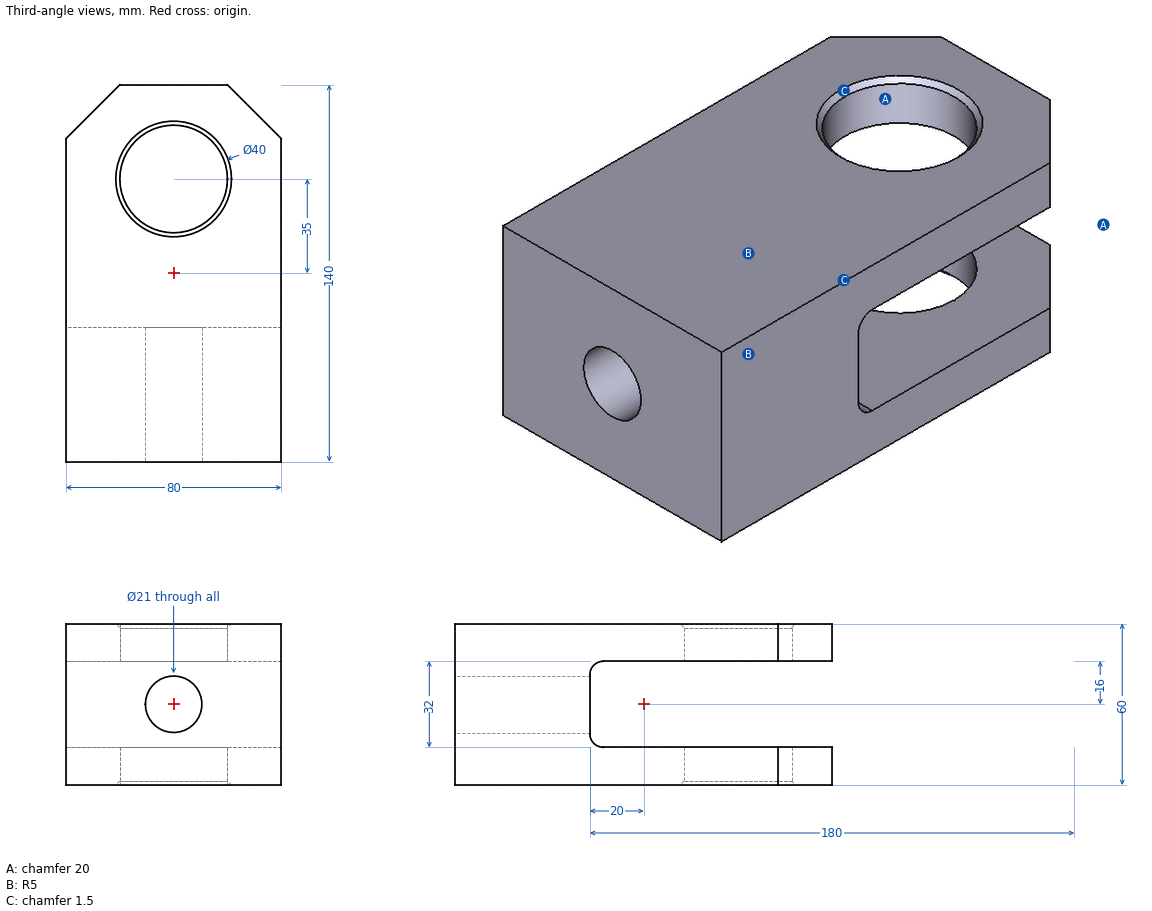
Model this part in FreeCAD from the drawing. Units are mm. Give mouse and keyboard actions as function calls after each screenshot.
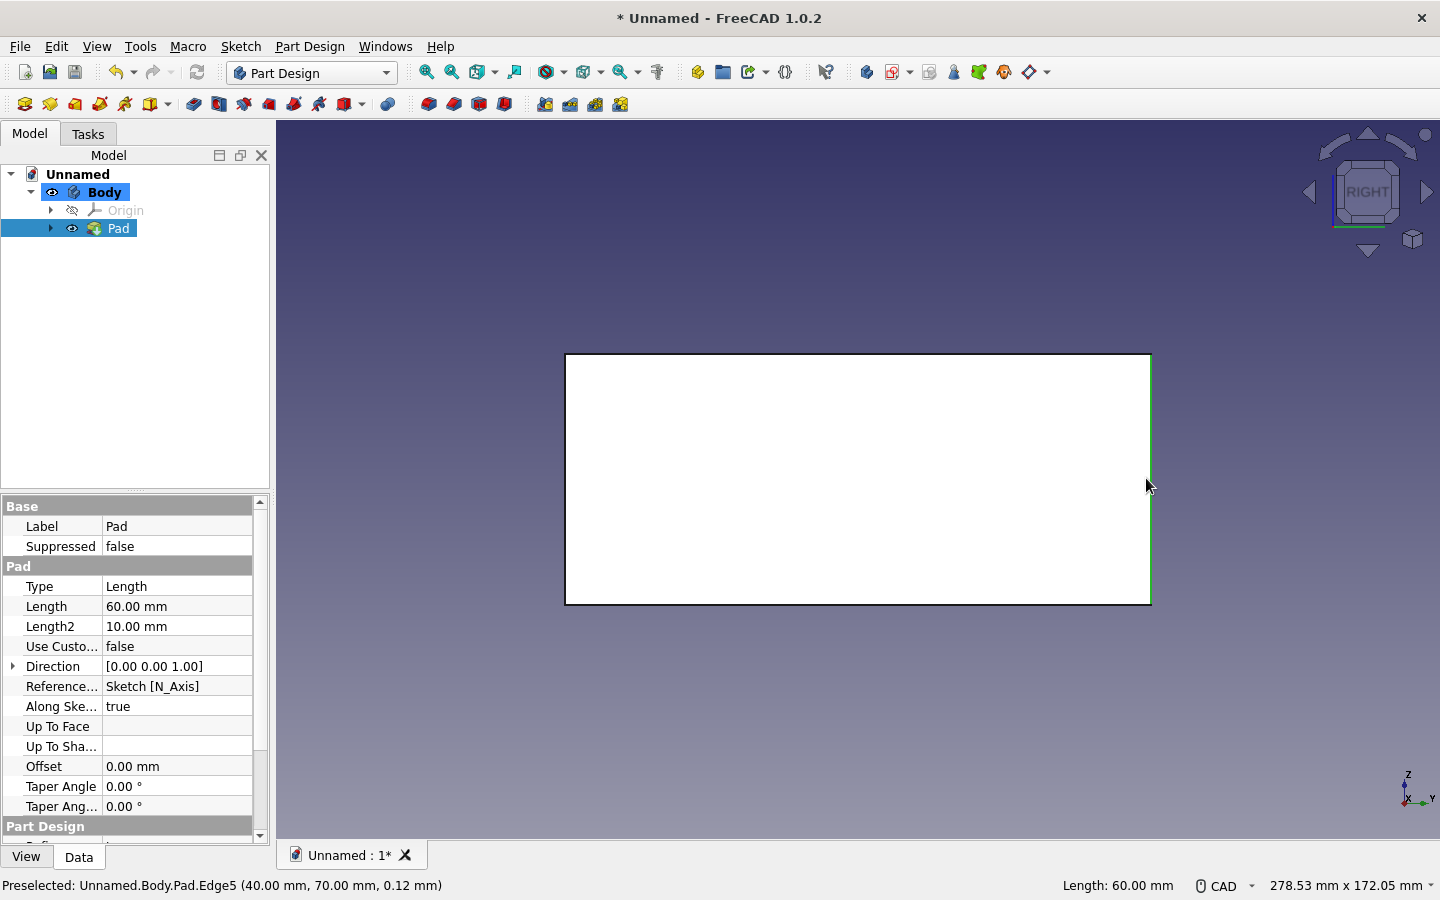
key(5)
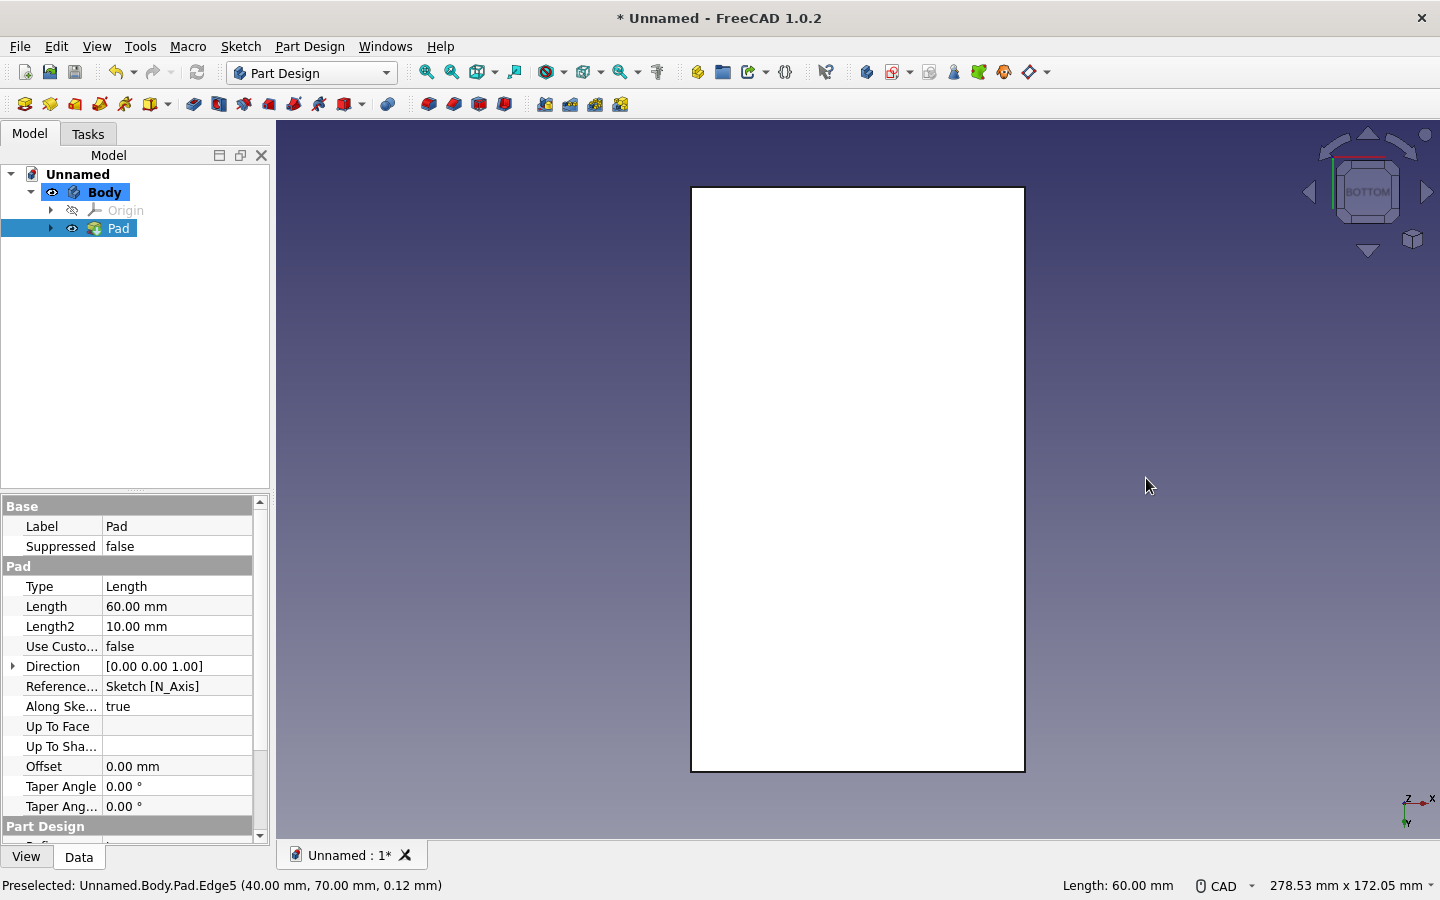
key(4)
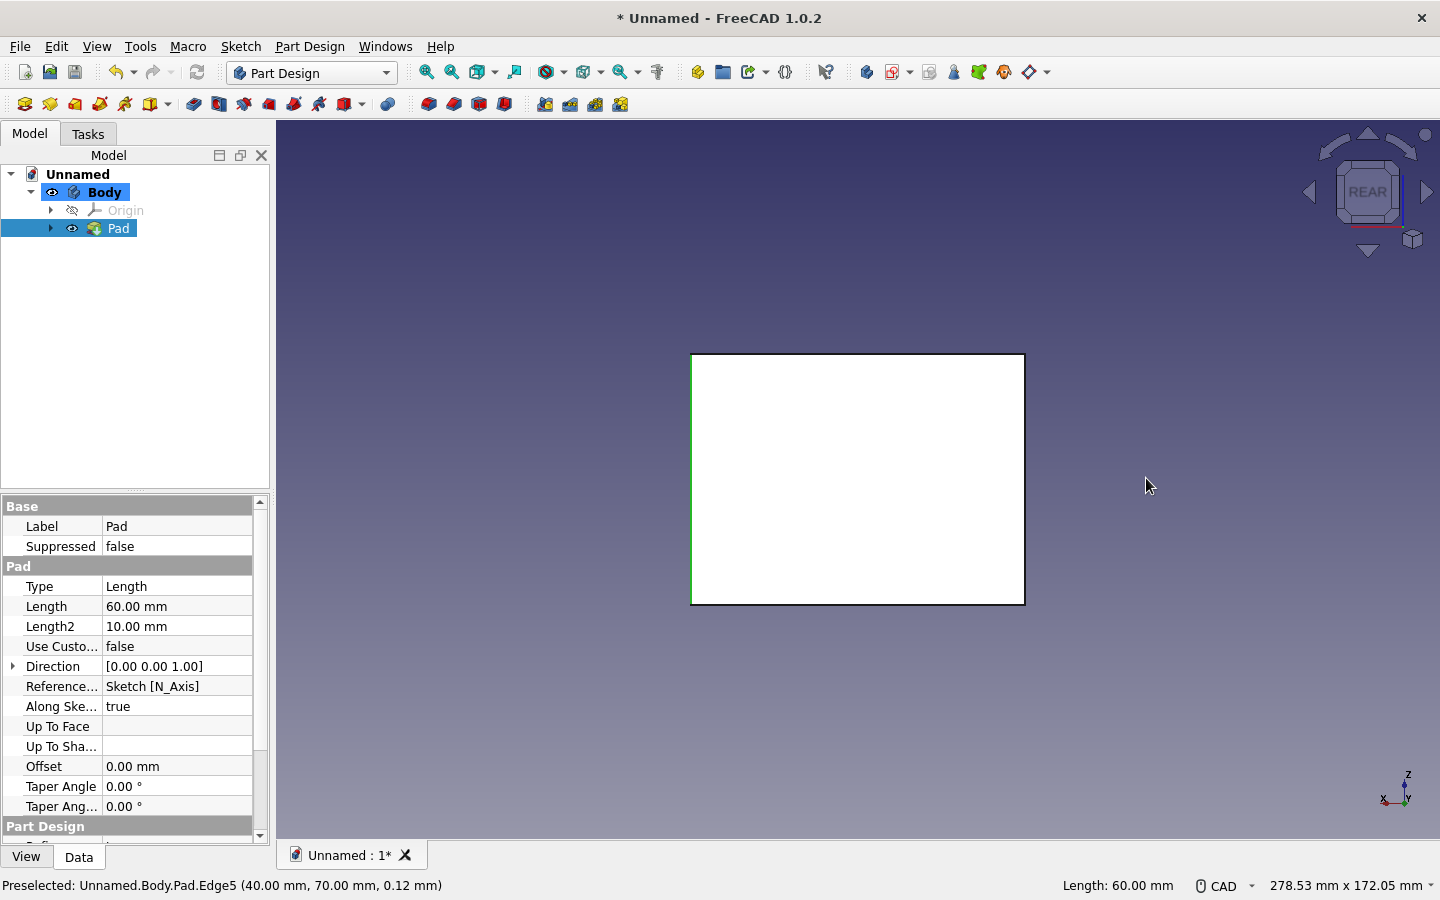
click(427, 72)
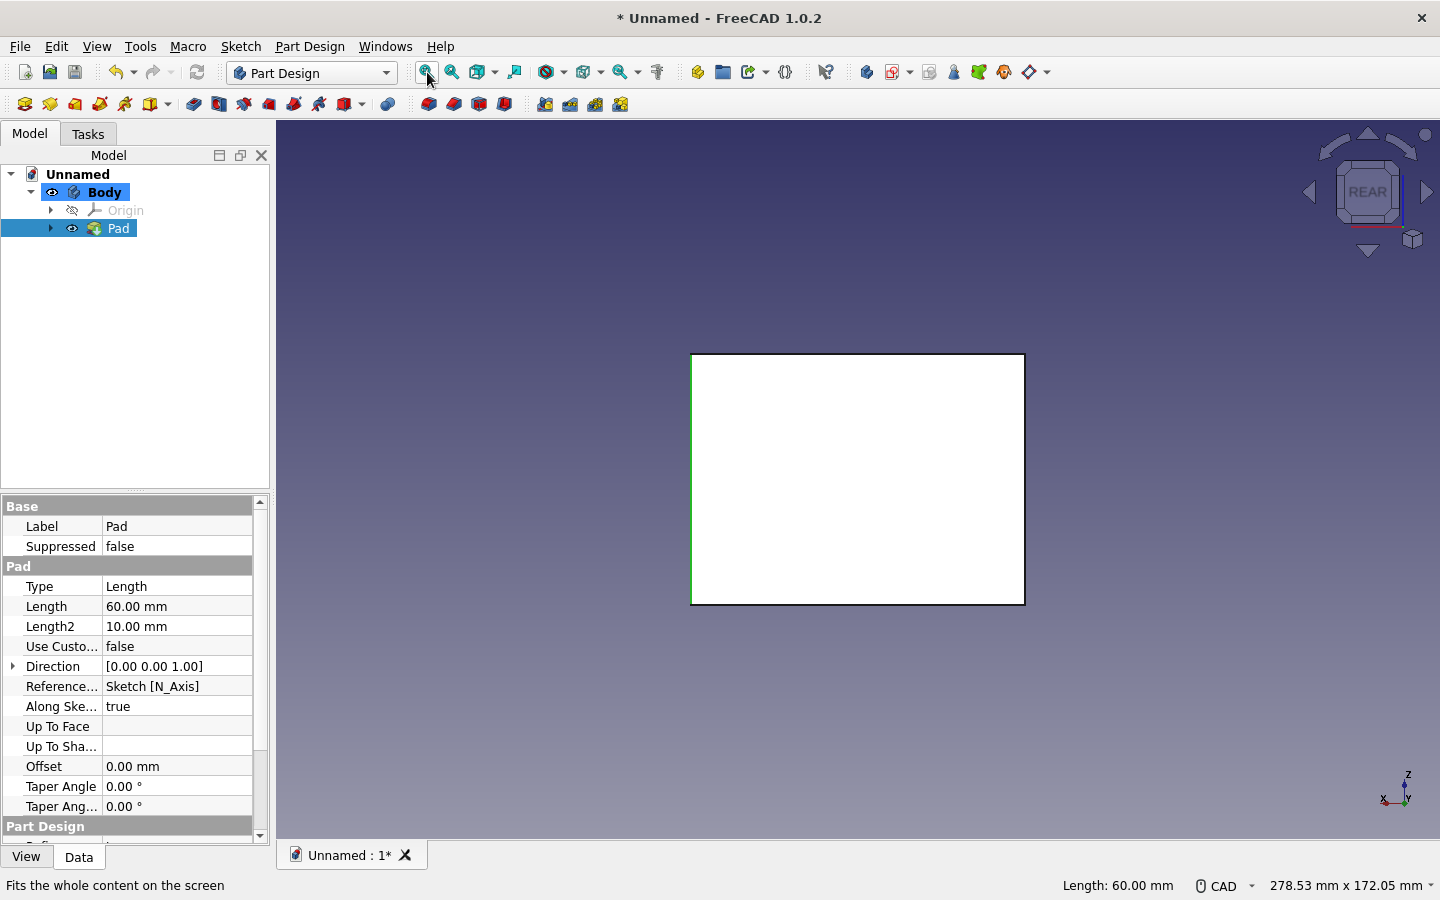
click(1025, 479, ctrl)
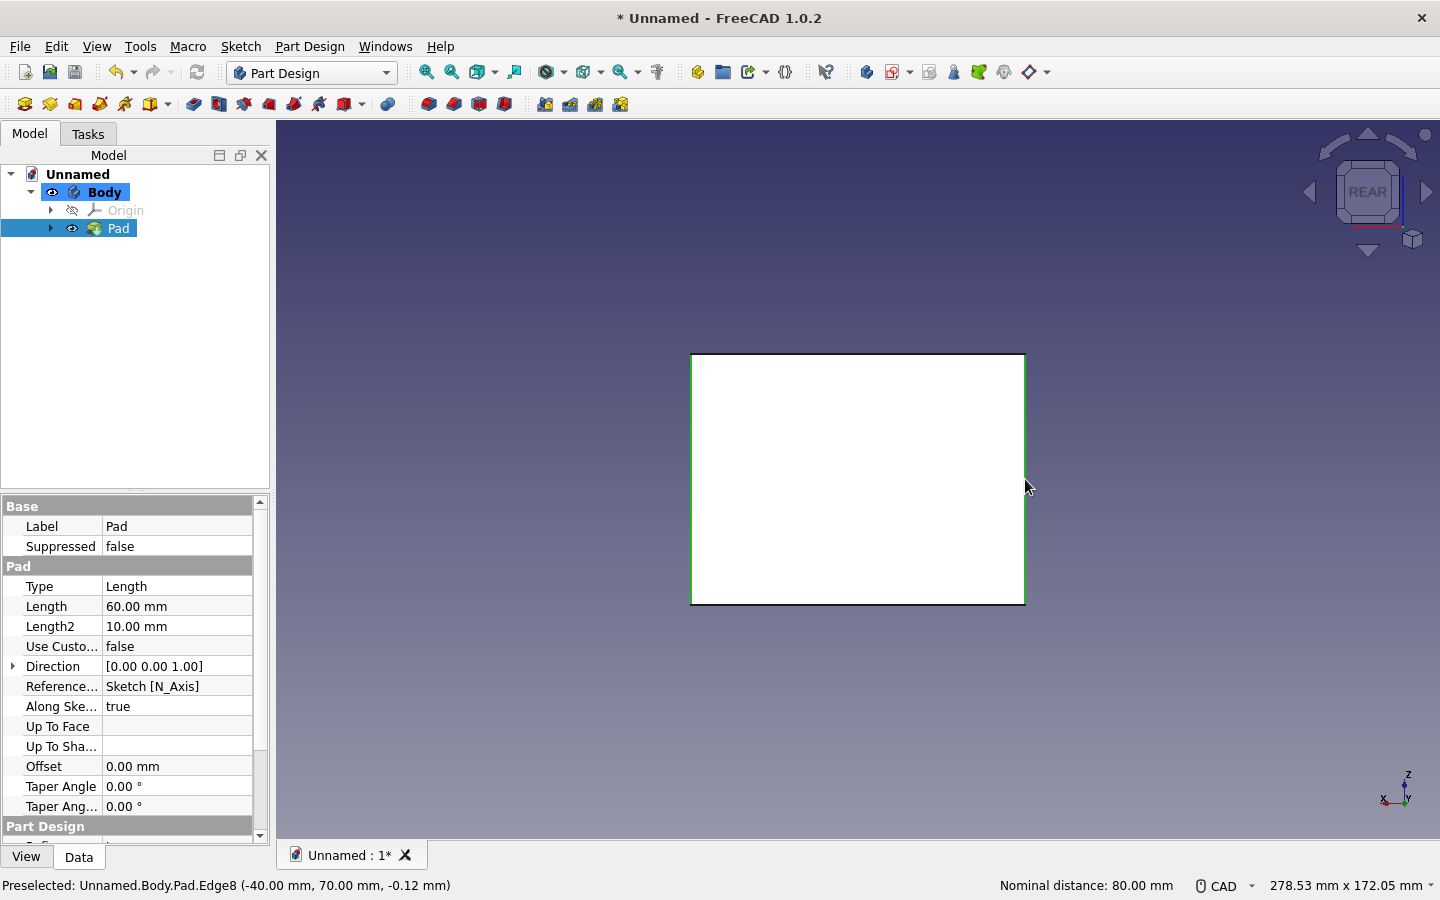
click(454, 104)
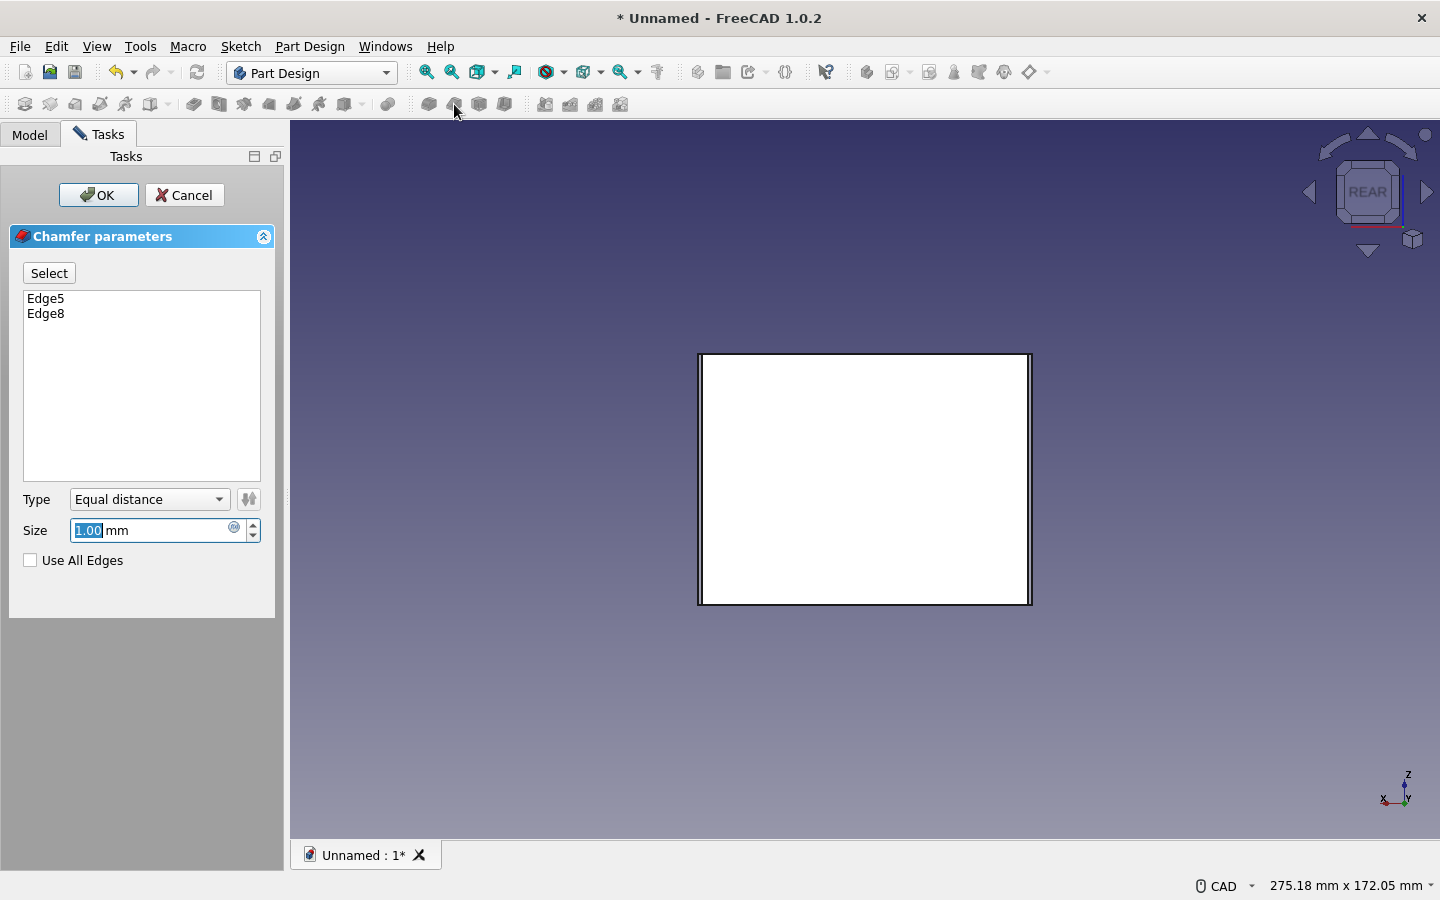
text(20)
key(Tab)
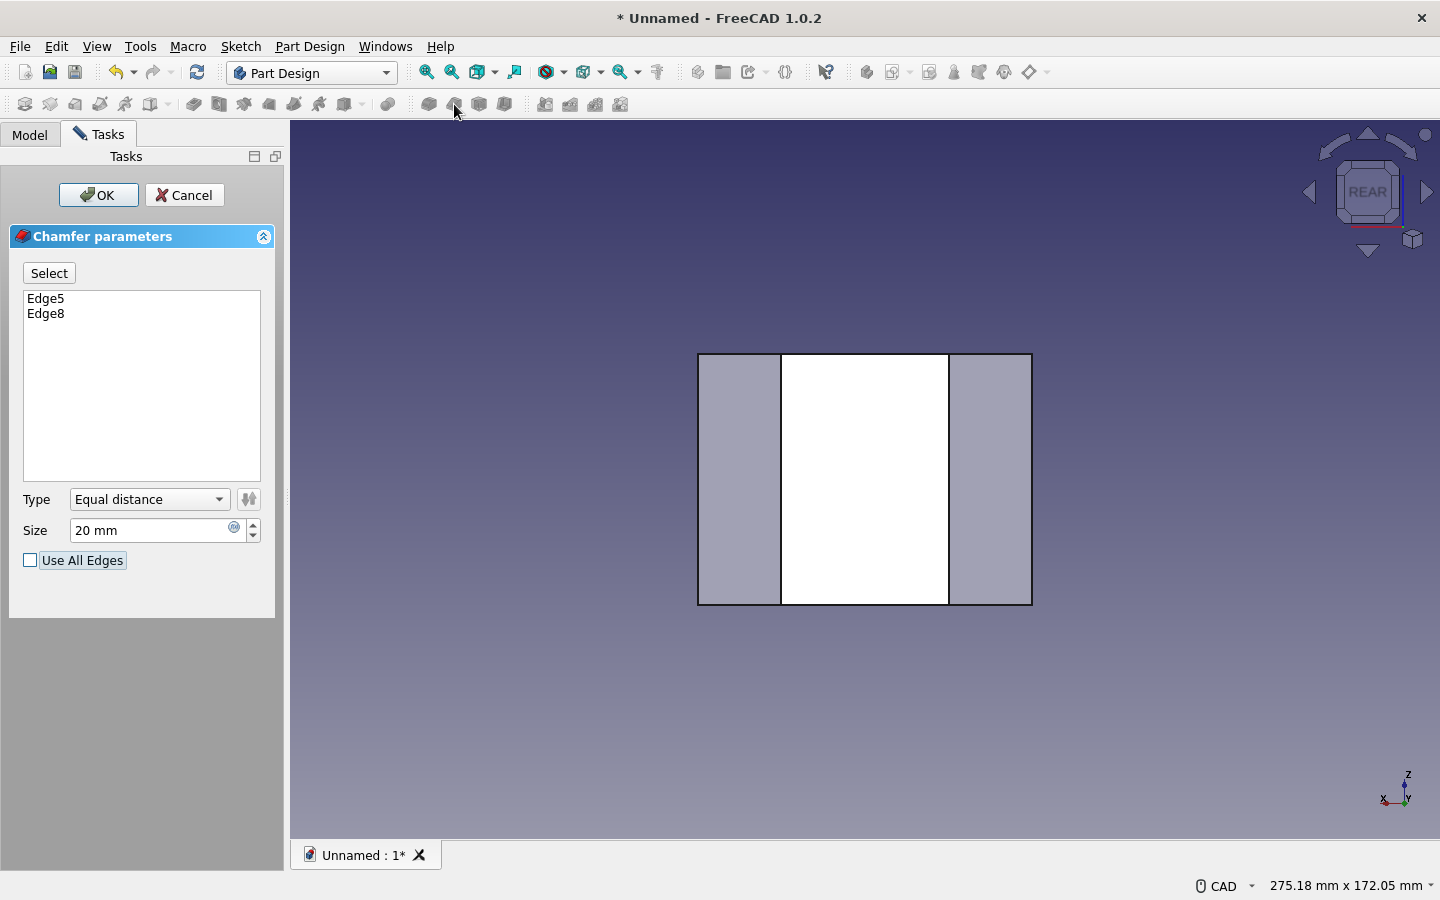
click(99, 195)